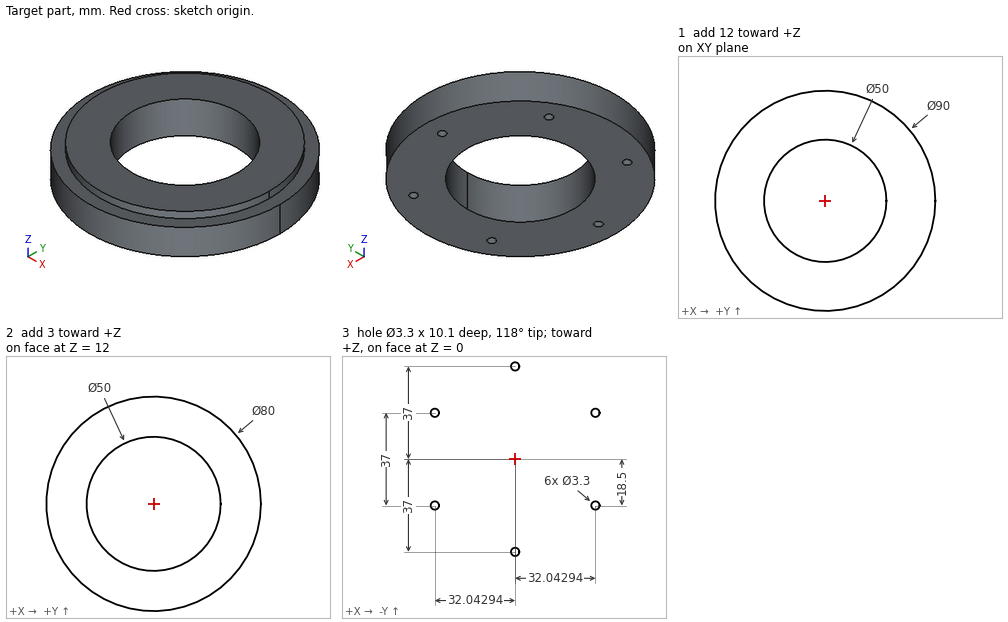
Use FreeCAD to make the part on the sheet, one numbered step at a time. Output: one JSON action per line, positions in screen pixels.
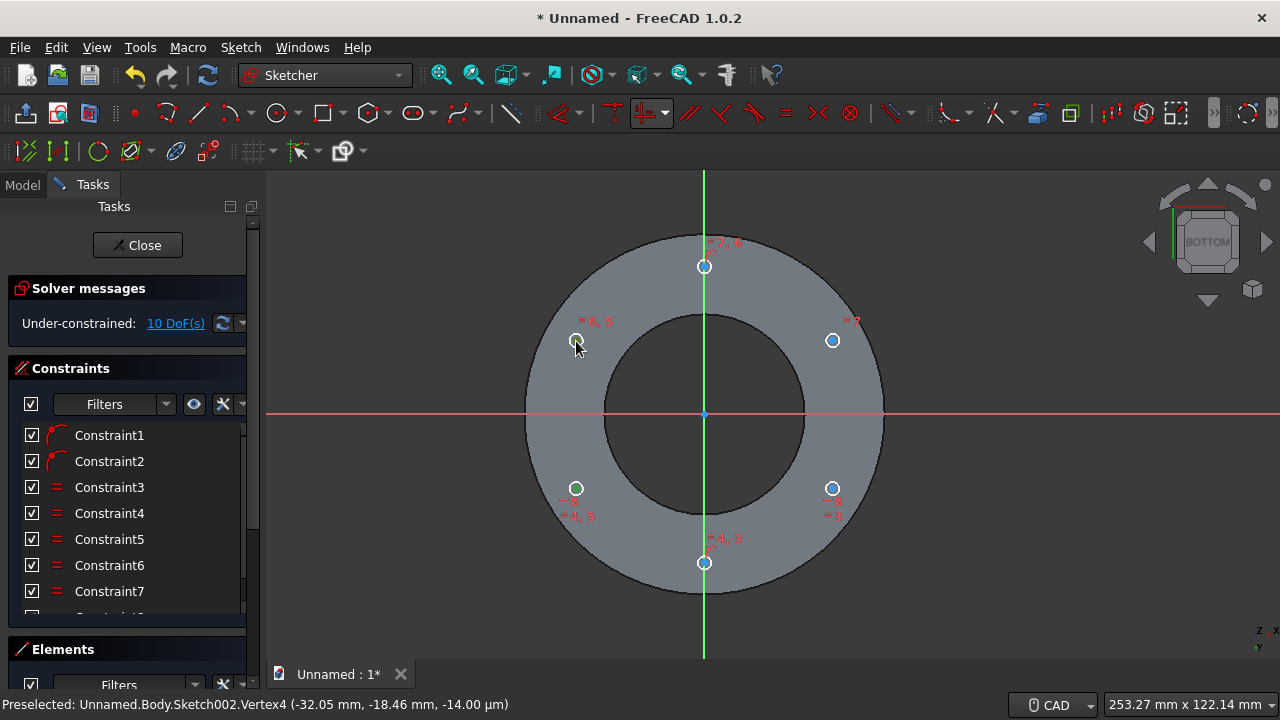
{"action": "key", "text": "v"}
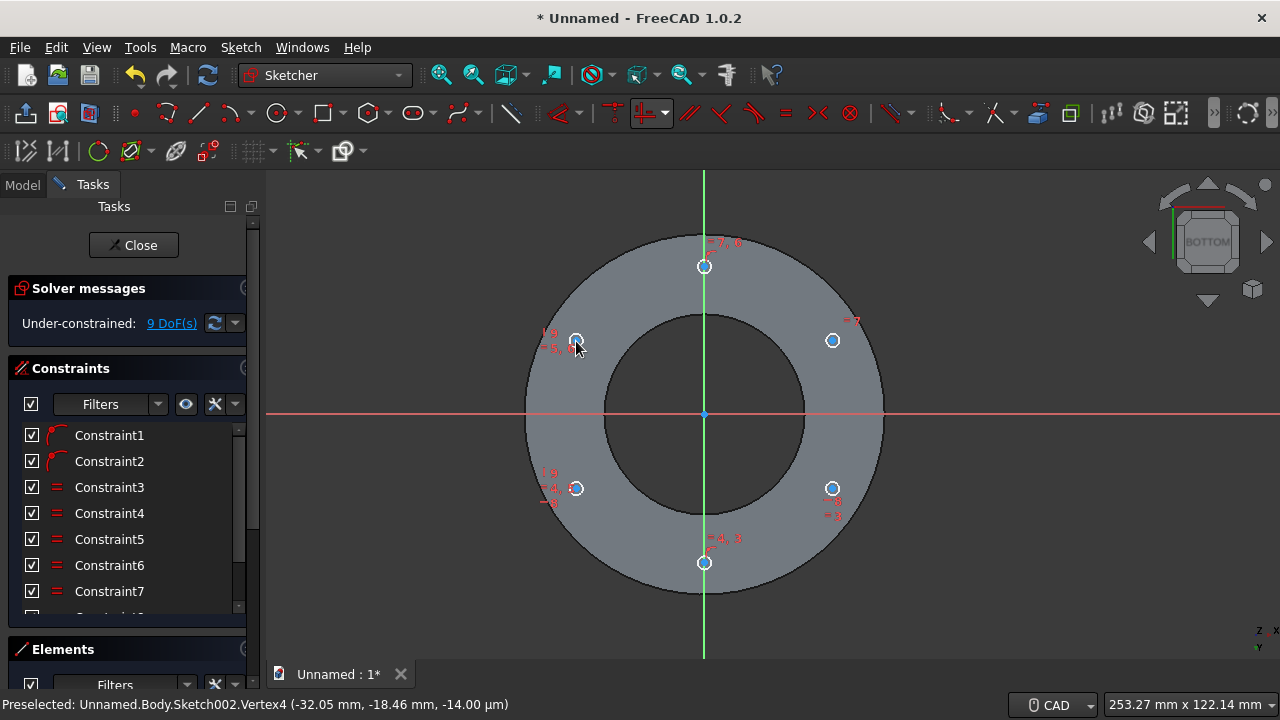
{"action": "left_click", "coordinate": [833, 489]}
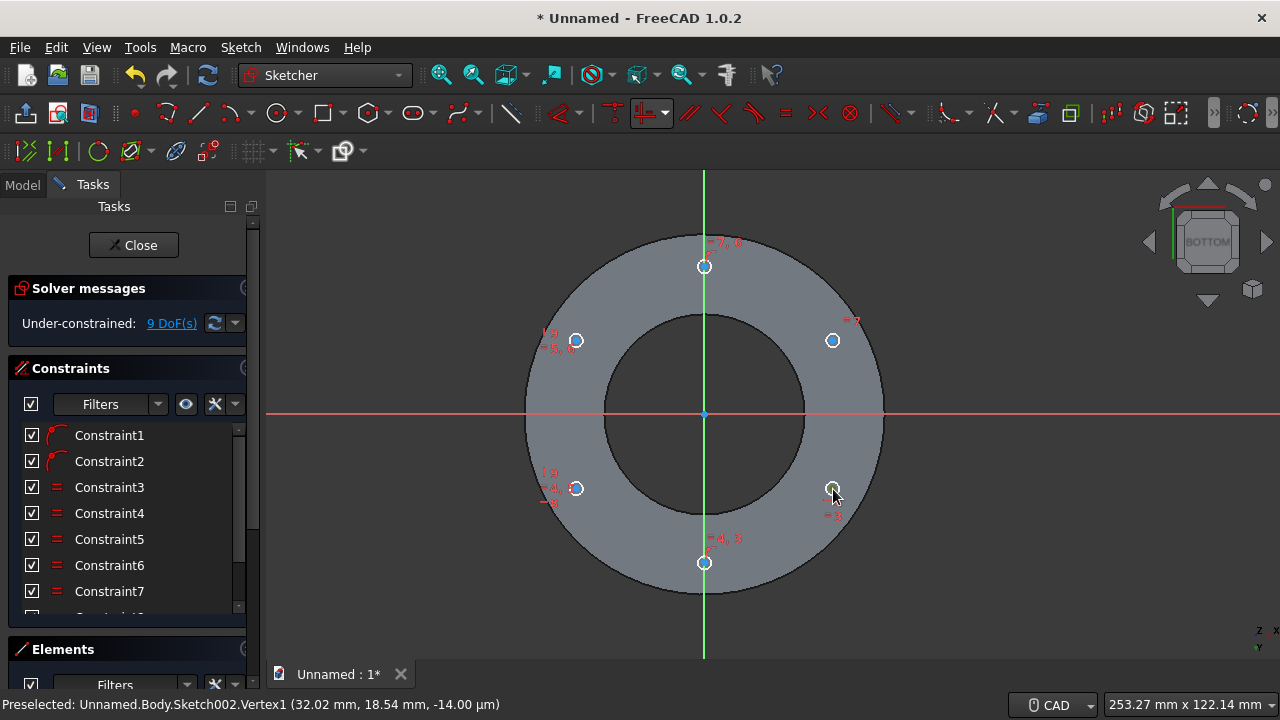
{"action": "left_click", "coordinate": [833, 341]}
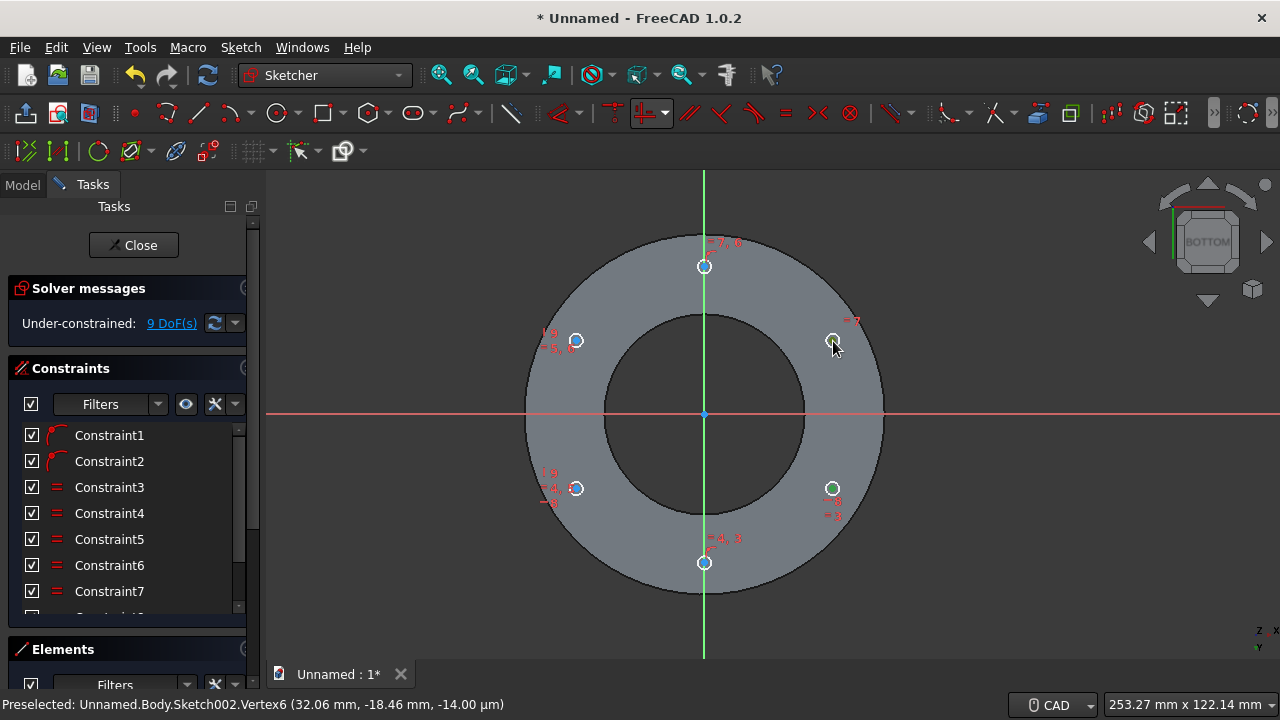
{"action": "key", "text": "v"}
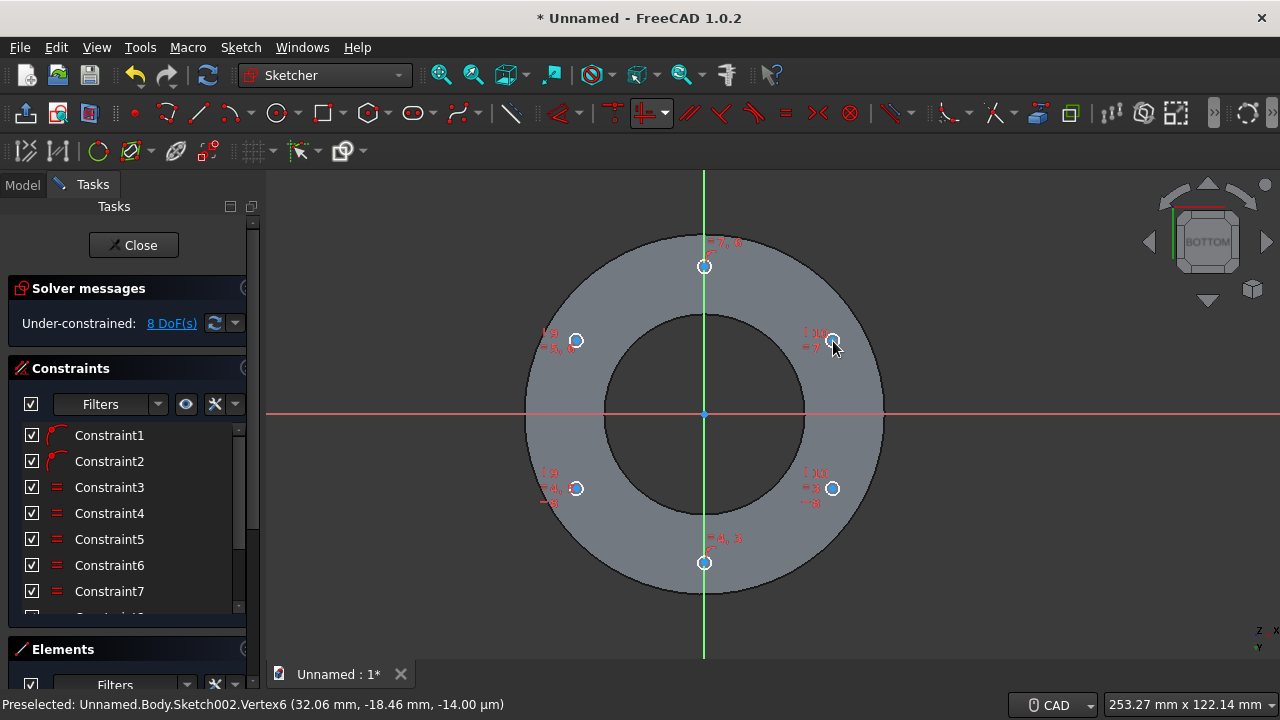
{"action": "left_click", "coordinate": [576, 341]}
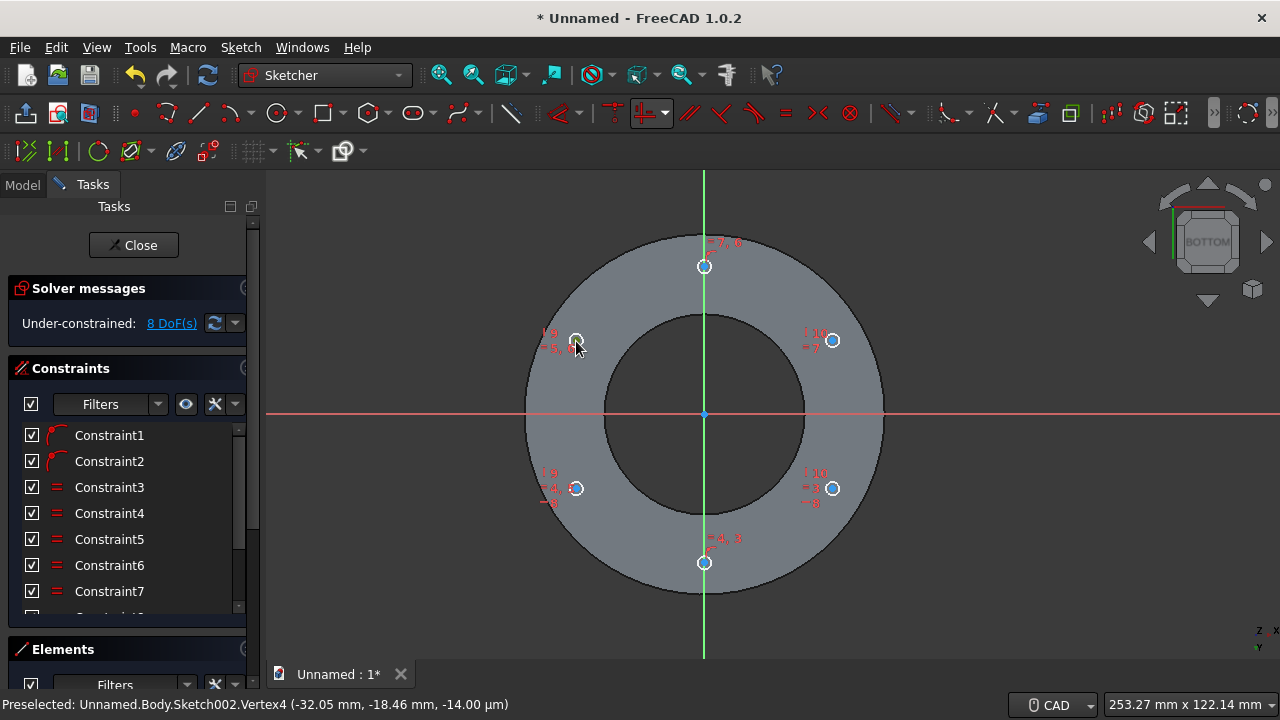
{"action": "left_click", "coordinate": [833, 341]}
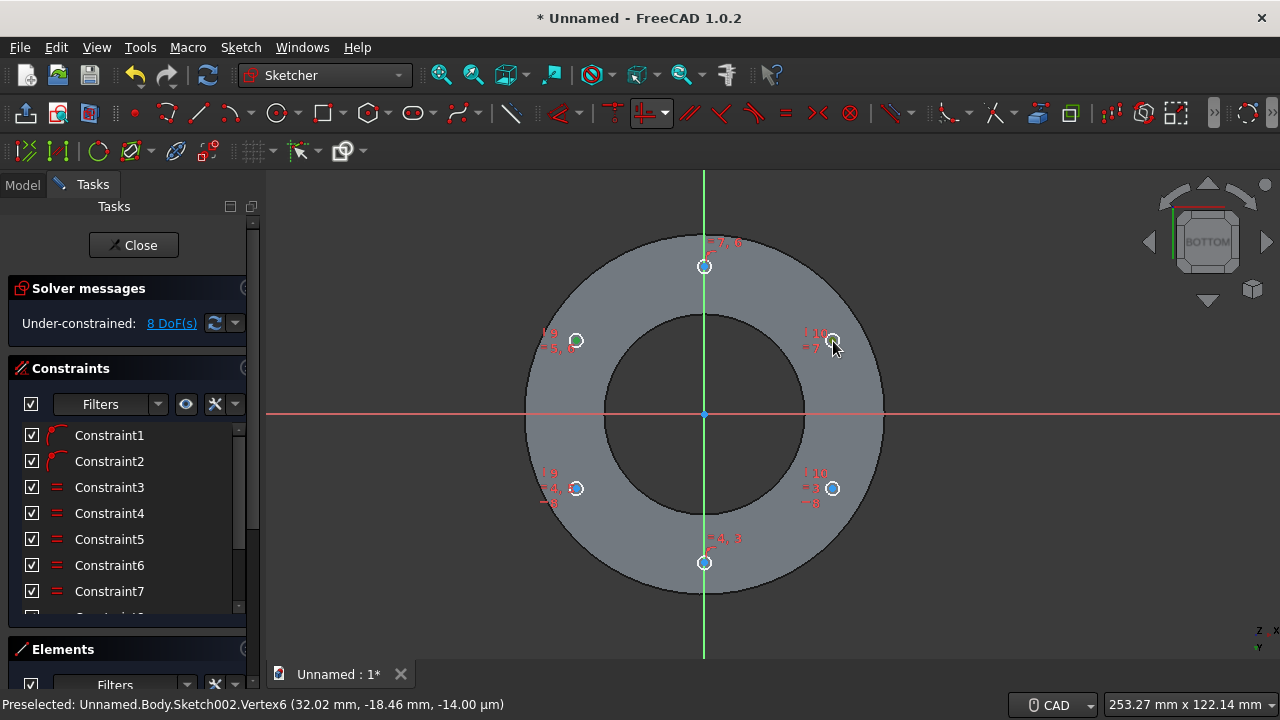
{"action": "left_click", "coordinate": [668, 114]}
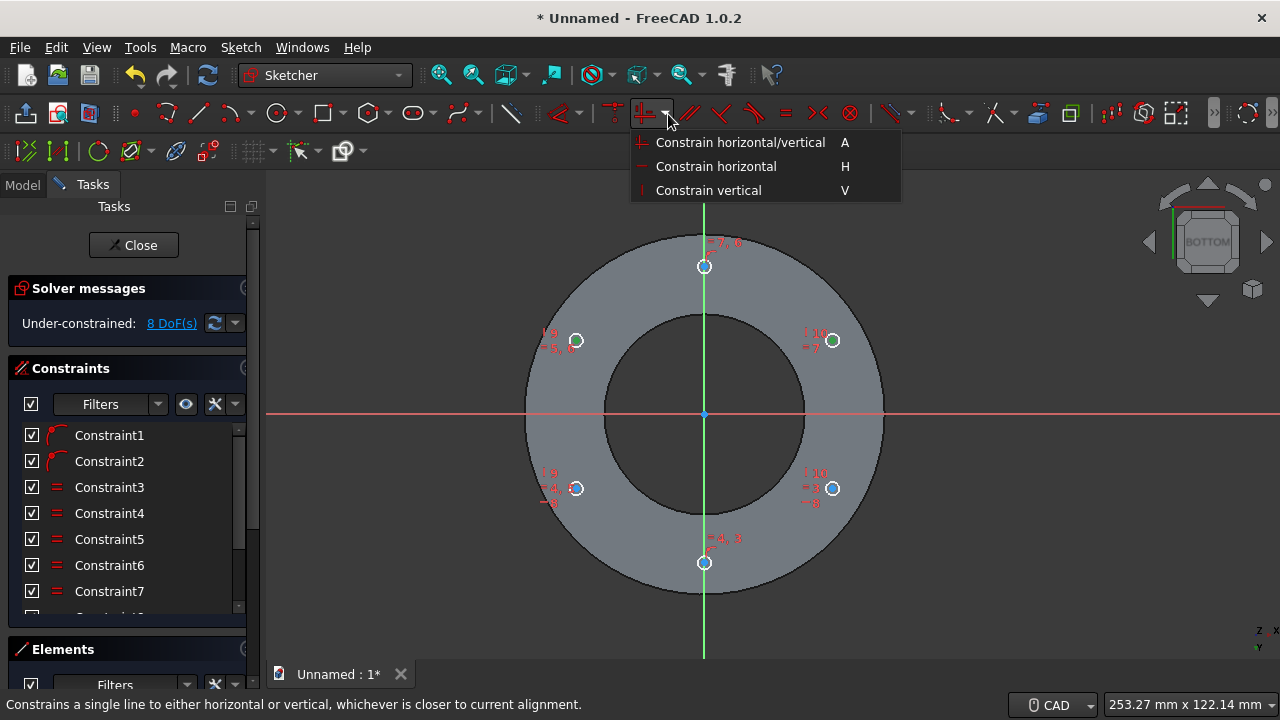
{"action": "left_click", "coordinate": [766, 166]}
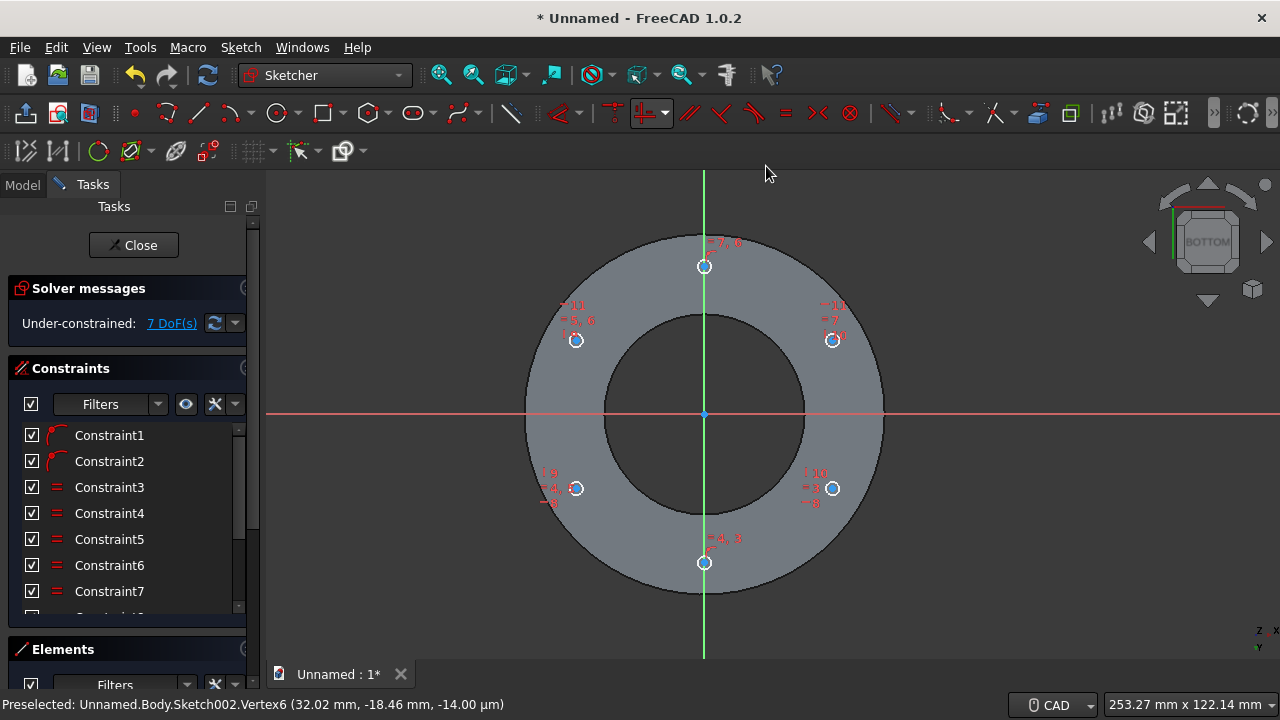
{"action": "left_click", "coordinate": [558, 114]}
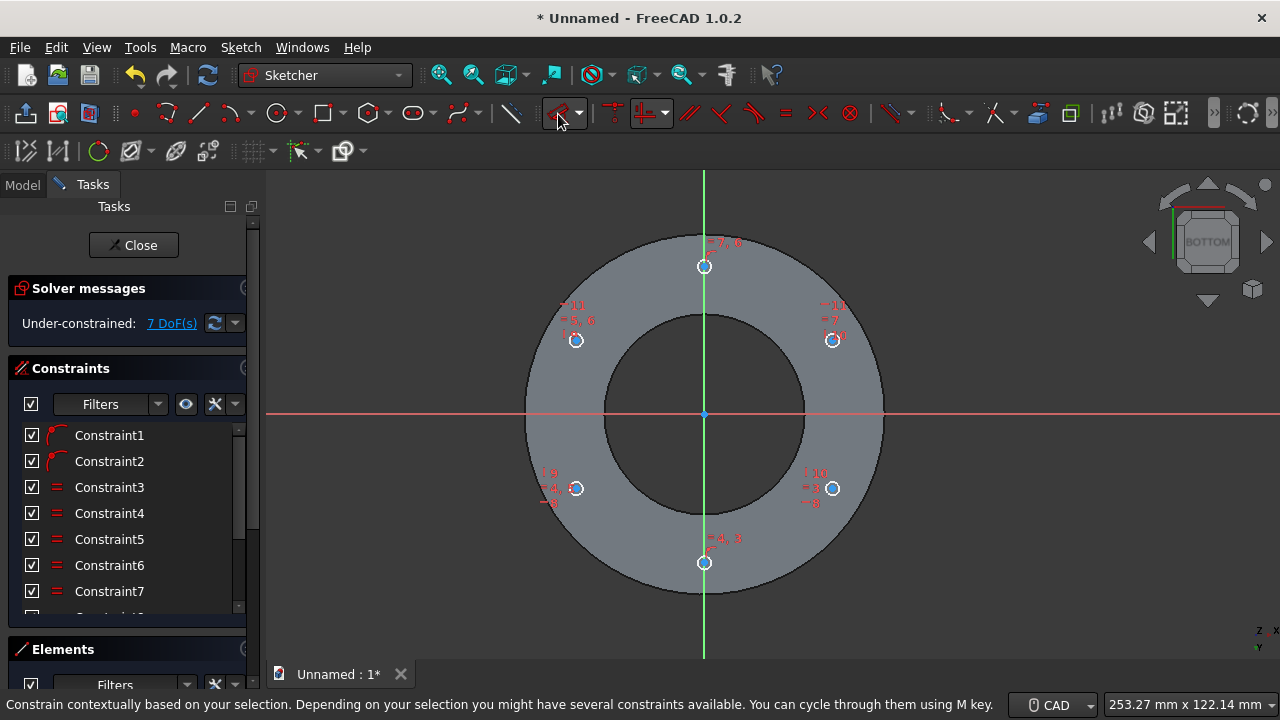
{"action": "scroll", "coordinate": [828, 484], "scroll_direction": "up", "scroll_amount": 6}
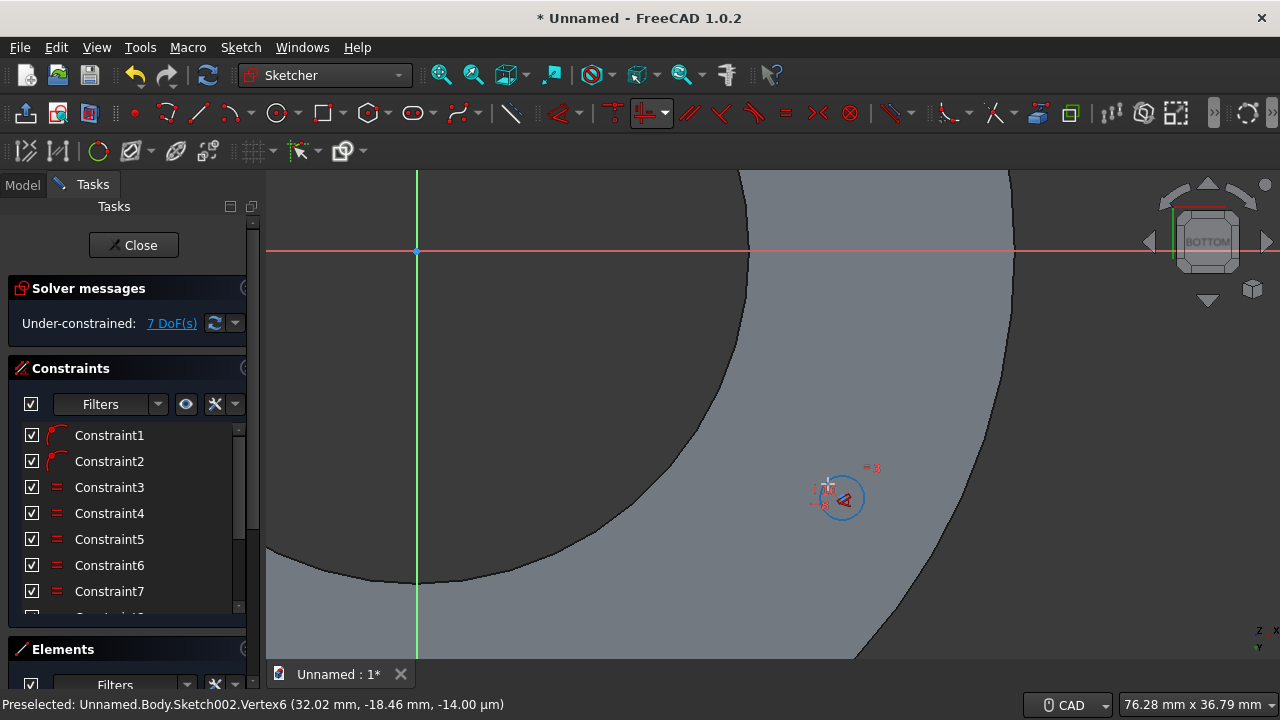
{"action": "left_click", "coordinate": [827, 482]}
{"action": "left_click", "coordinate": [805, 459]}